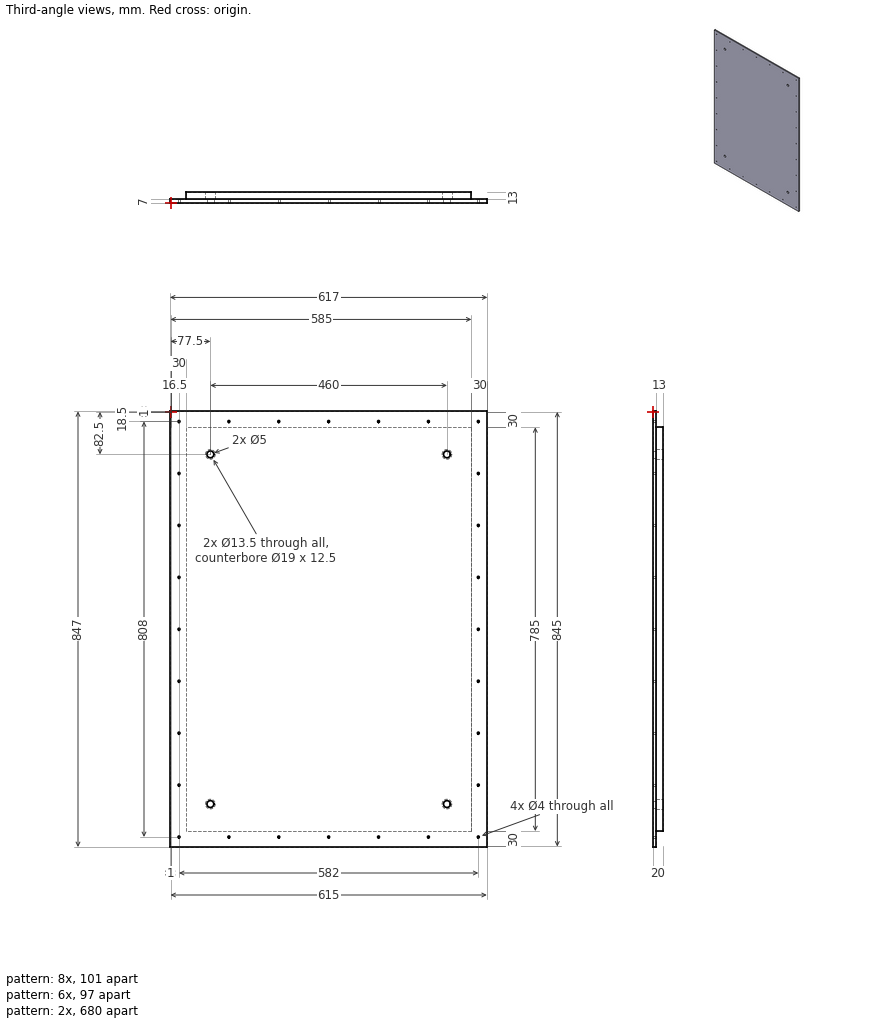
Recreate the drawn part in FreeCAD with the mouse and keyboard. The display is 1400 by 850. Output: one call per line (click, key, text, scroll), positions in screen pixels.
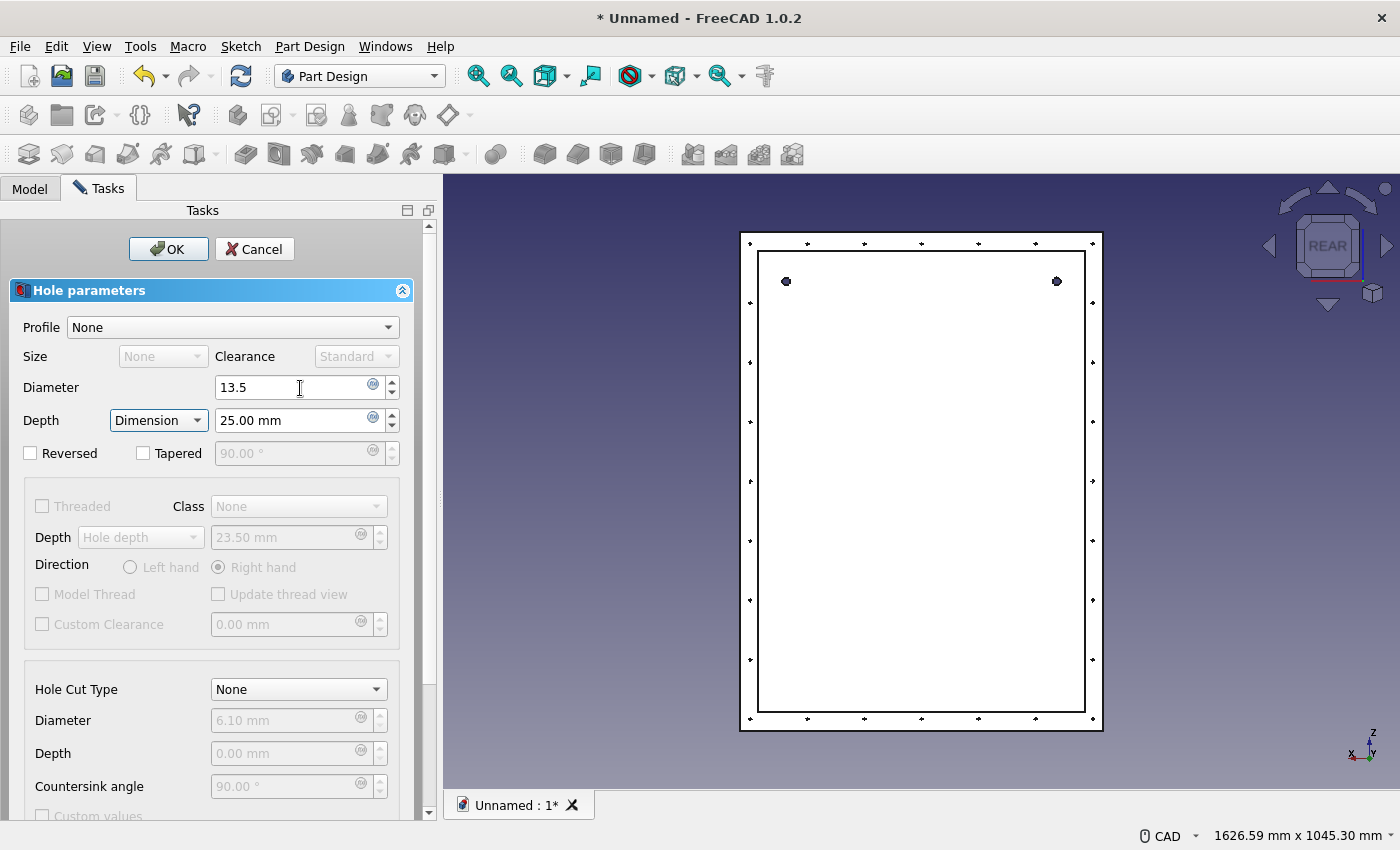
click(160, 420)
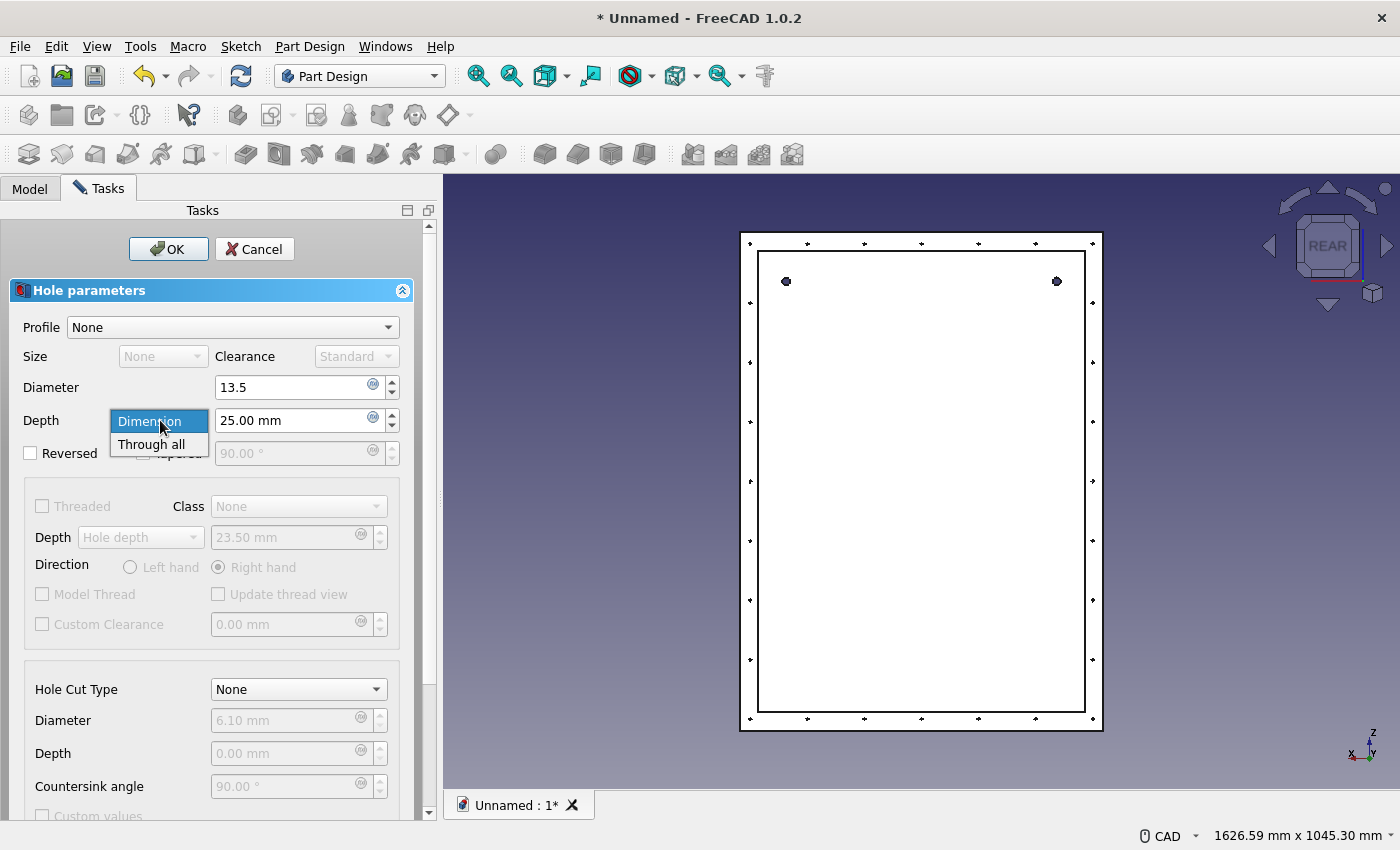
click(158, 444)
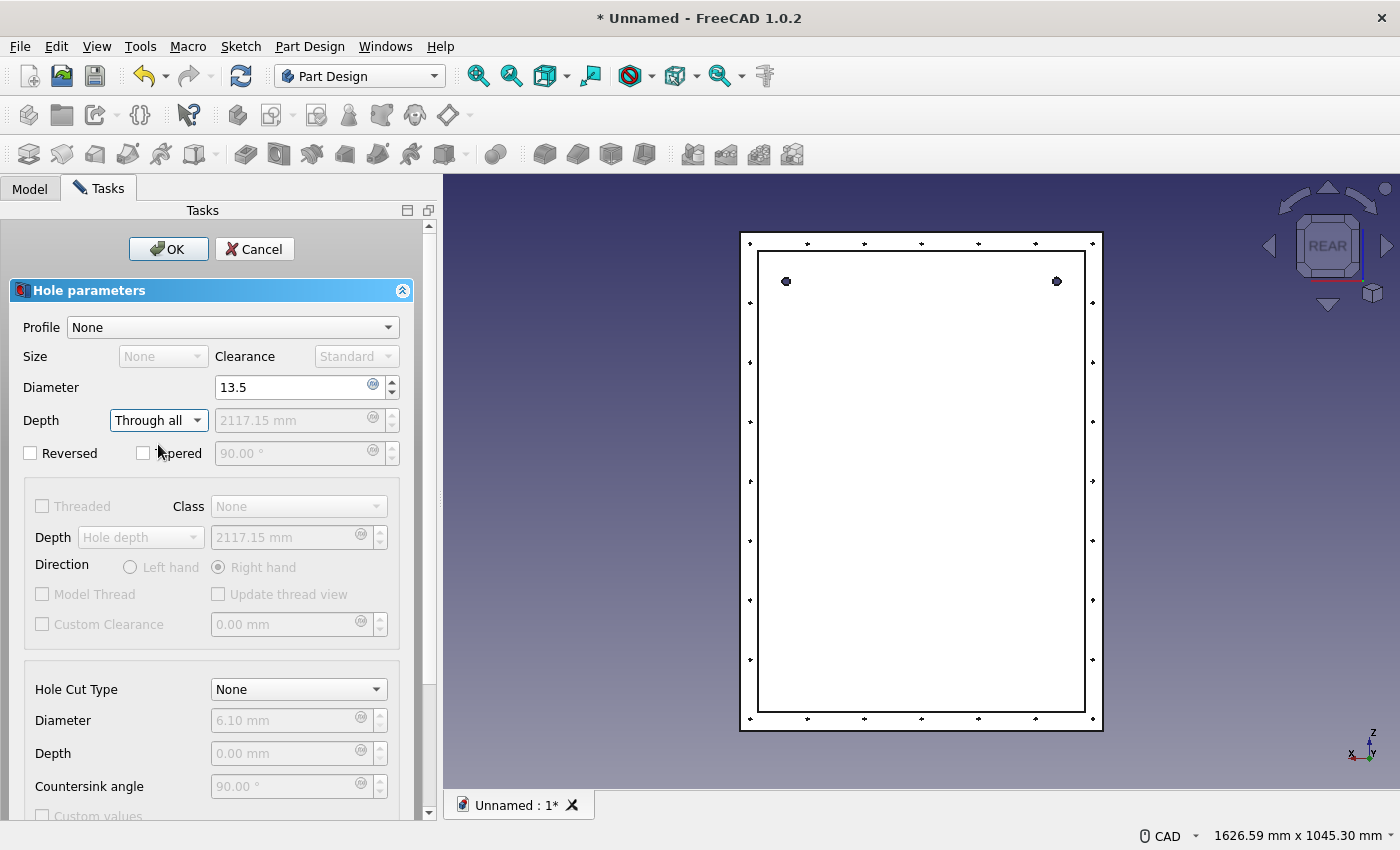
click(300, 690)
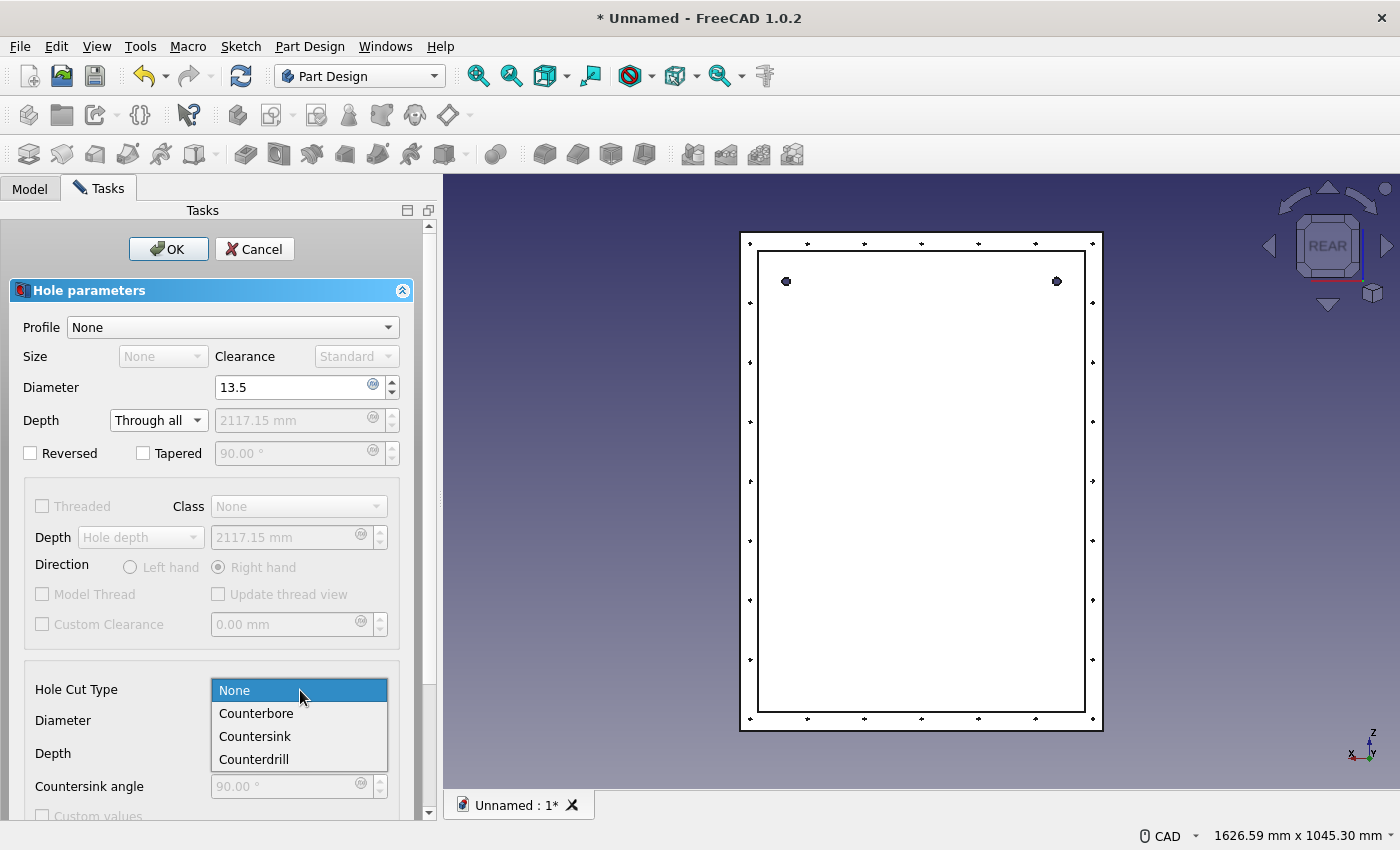
click(298, 714)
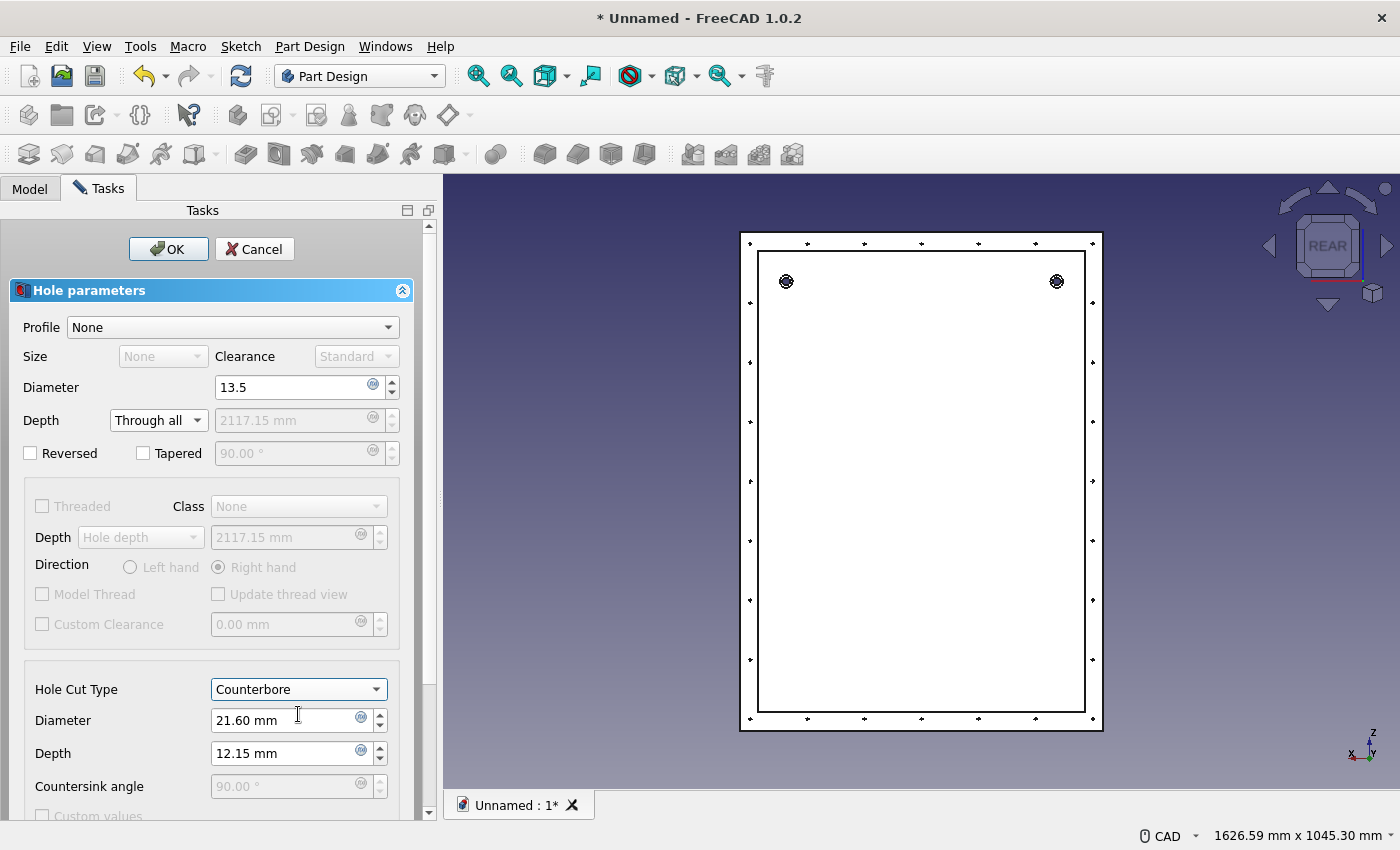
triple_click(292, 720)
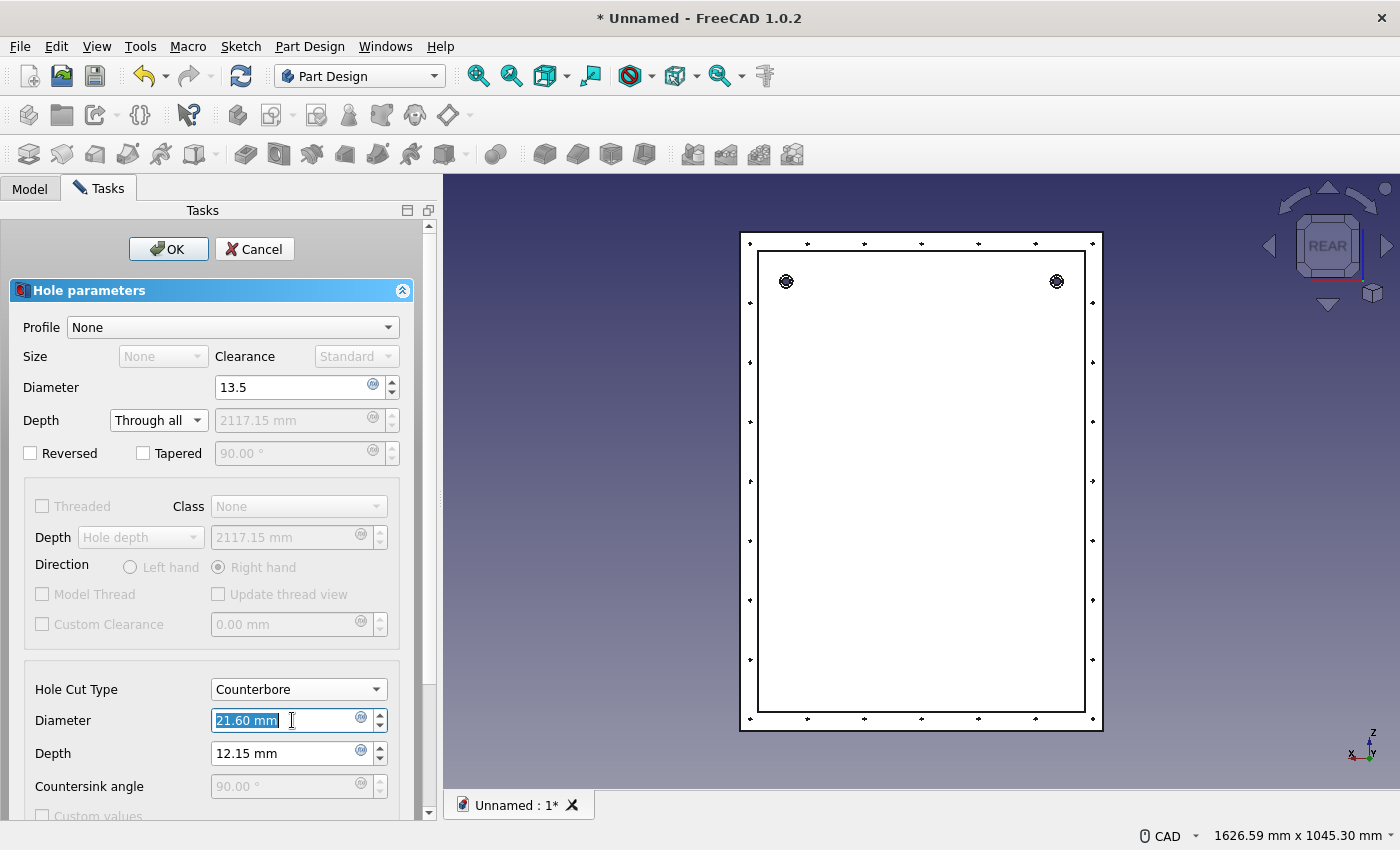
text(19)
key(Tab)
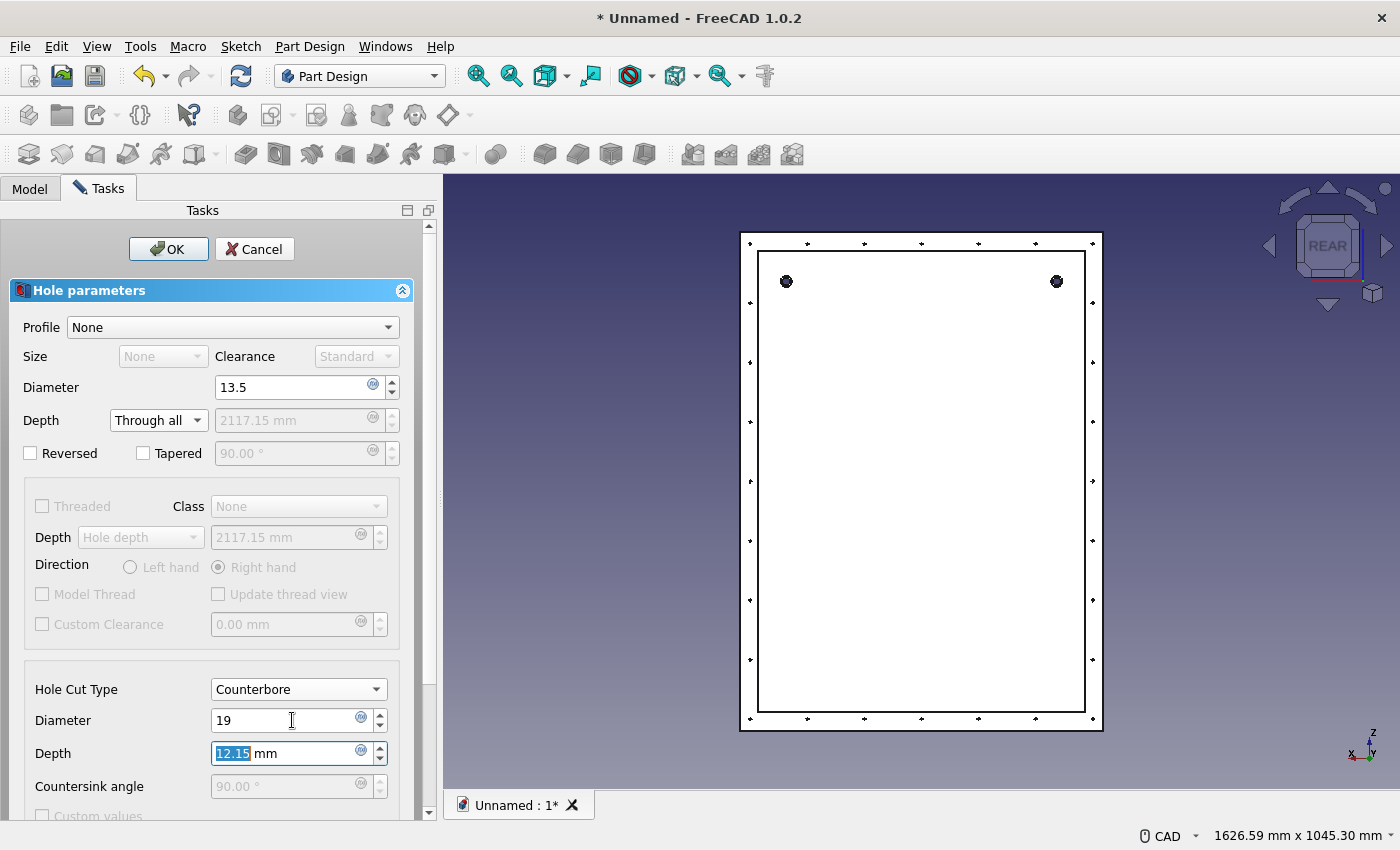
text(12.5)
key(Tab)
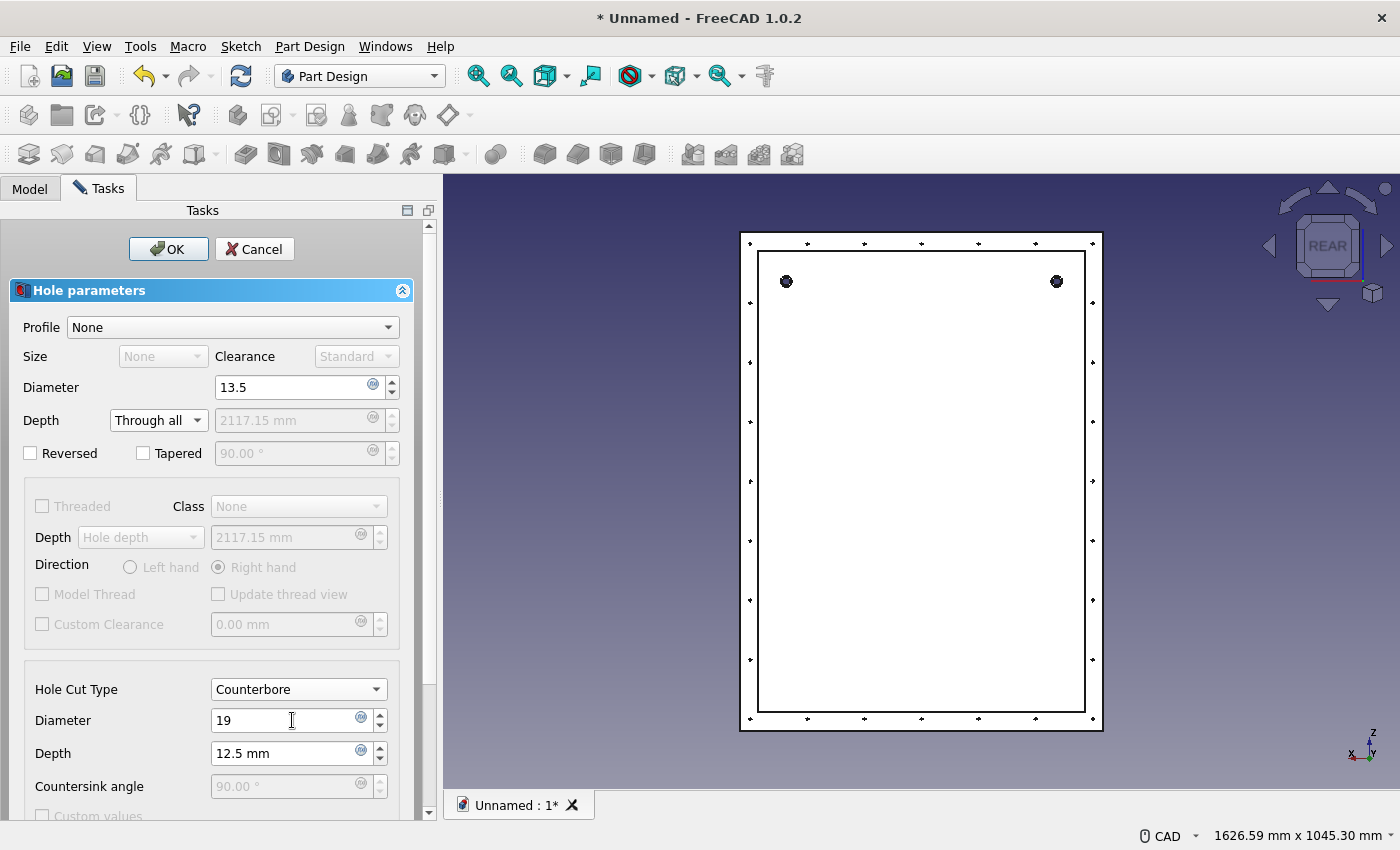
click(169, 249)